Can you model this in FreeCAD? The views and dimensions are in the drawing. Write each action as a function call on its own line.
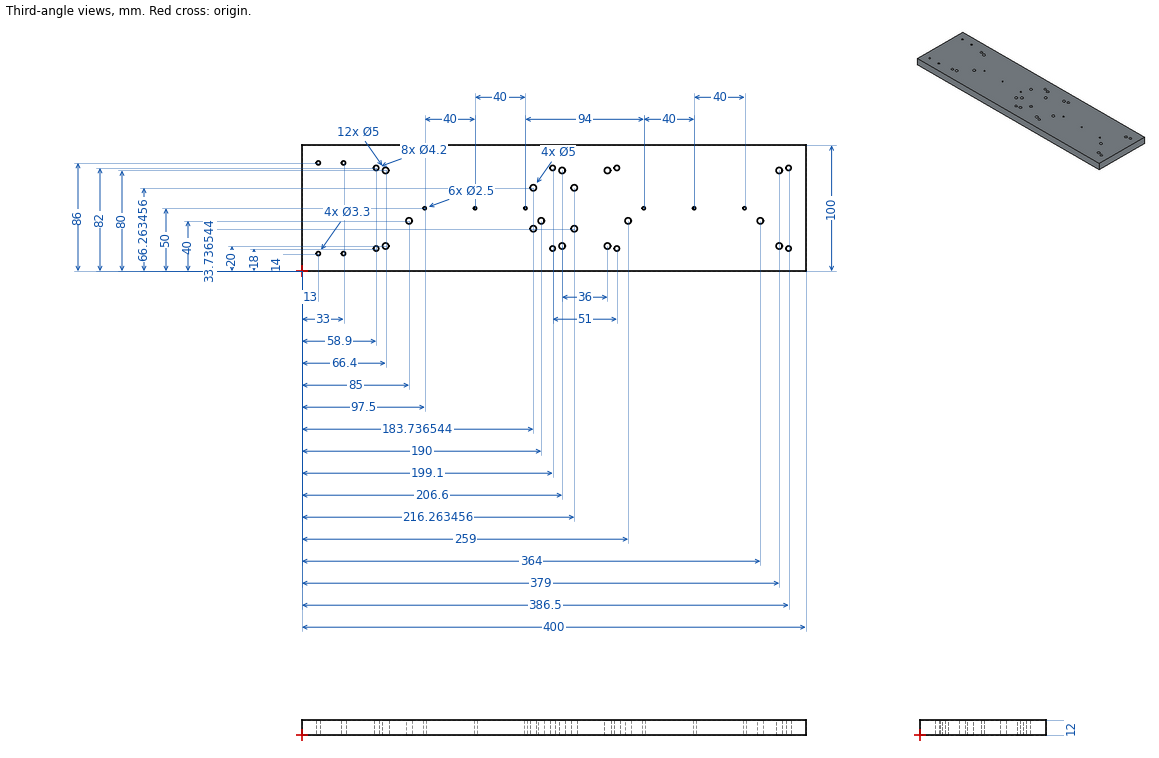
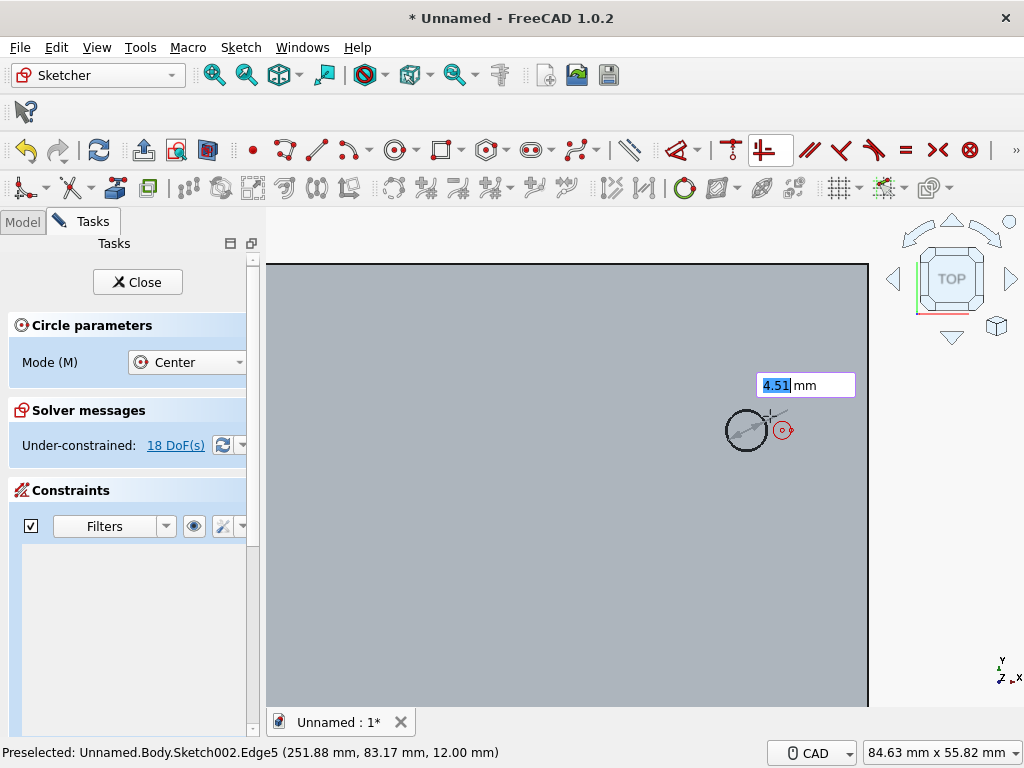
click(761, 411)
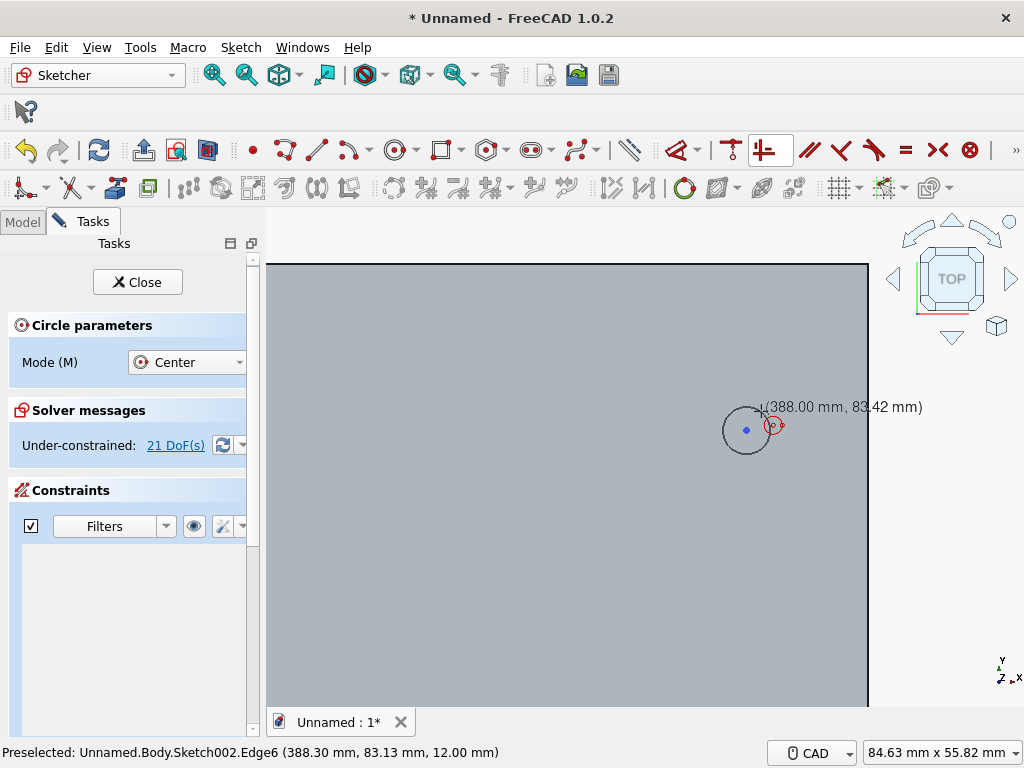
scroll(770, 416, down, 11)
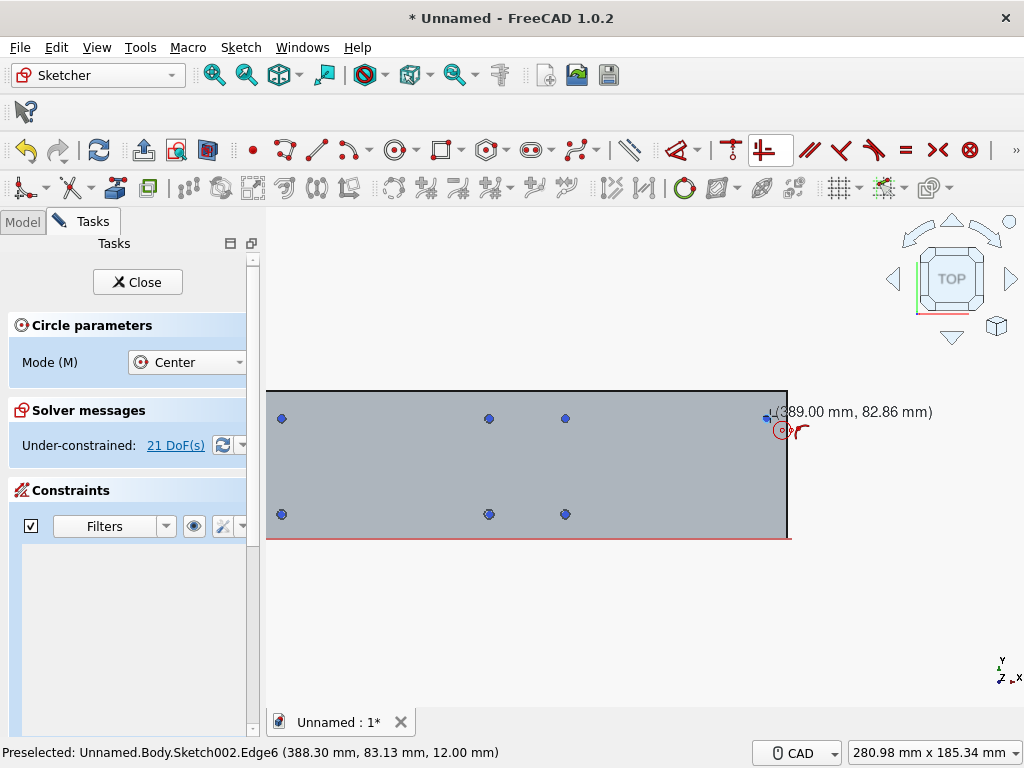
scroll(768, 481, up, 12)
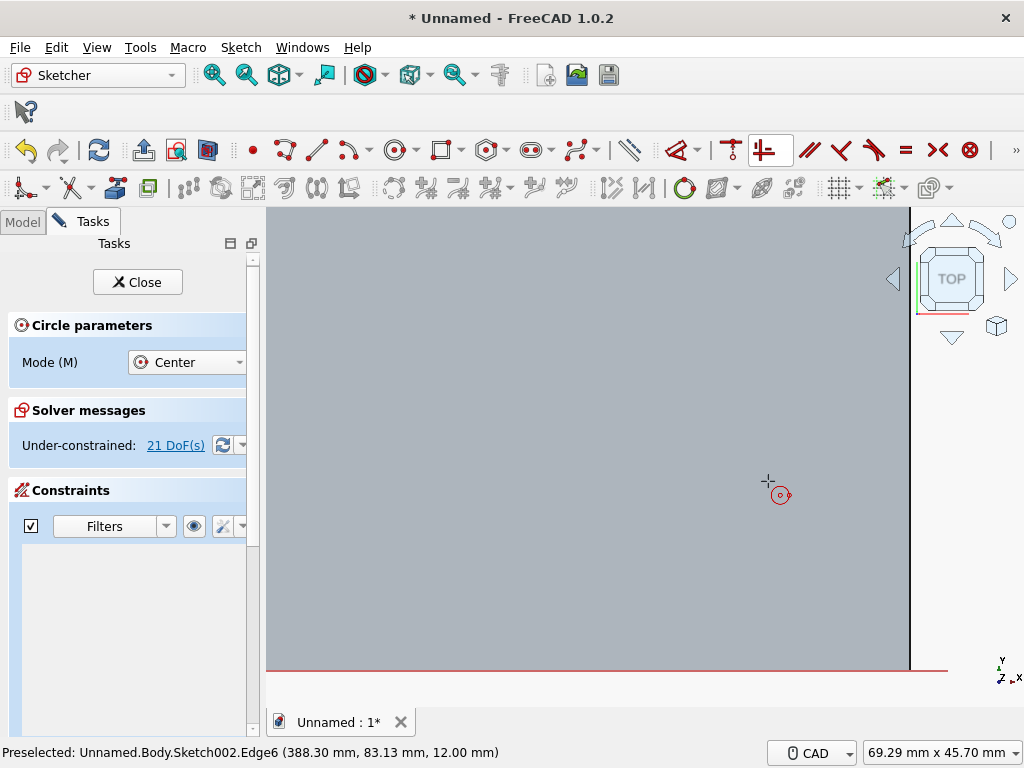
scroll(768, 482, down, 12)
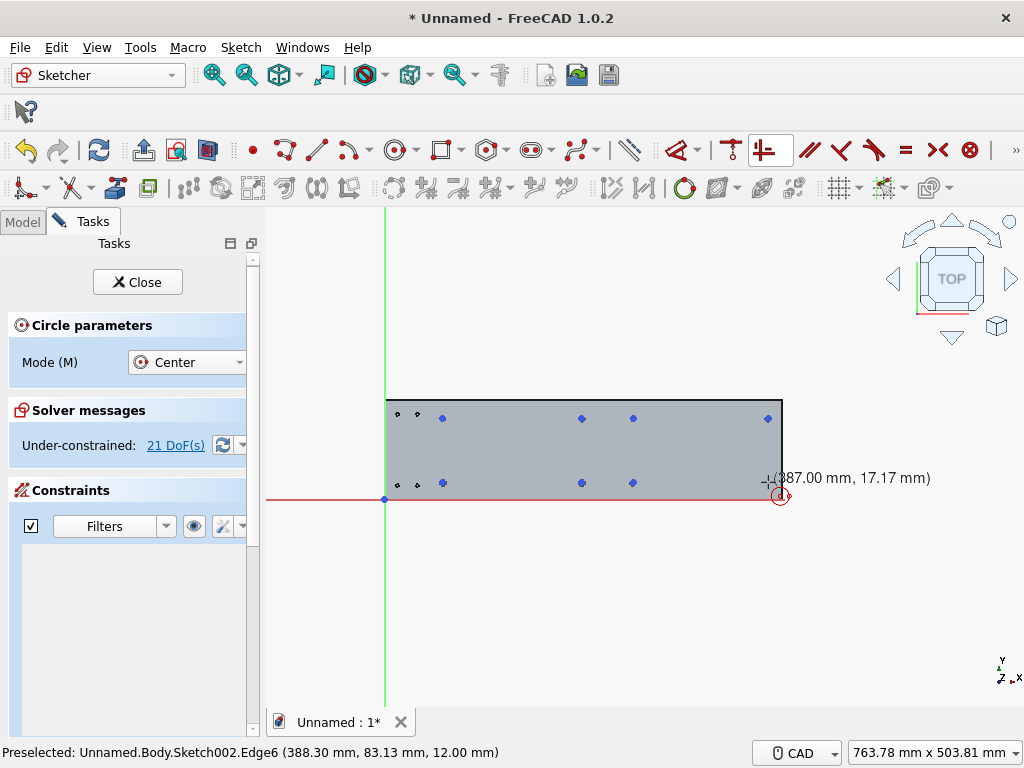
click(768, 482)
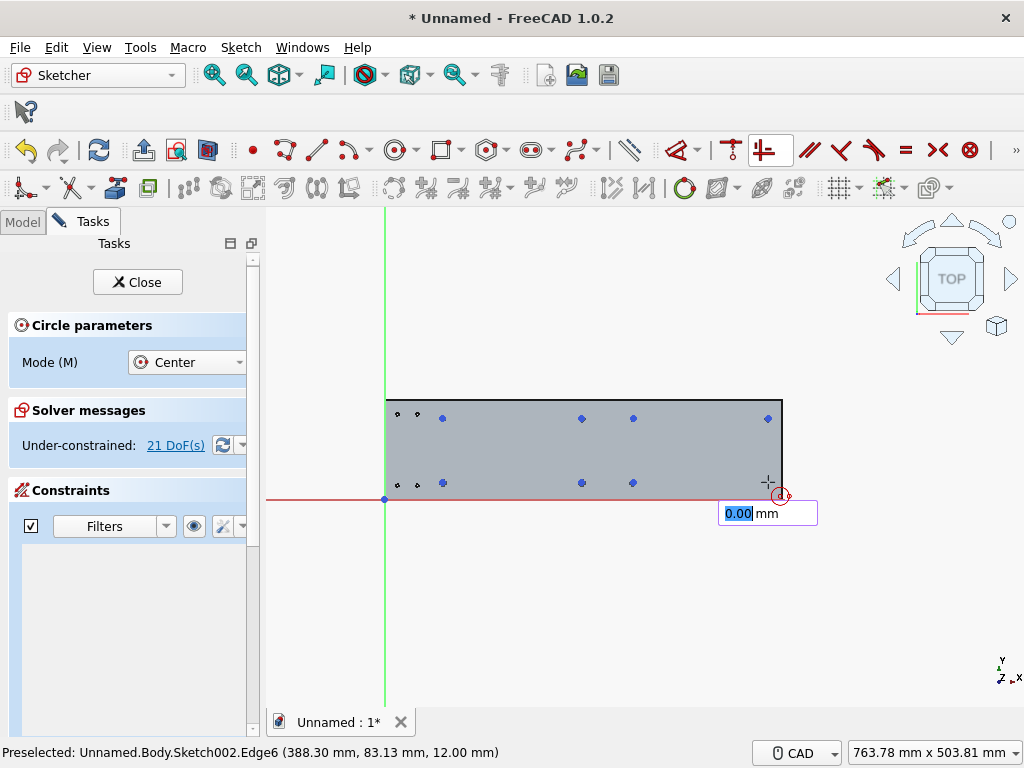
scroll(770, 480, up, 11)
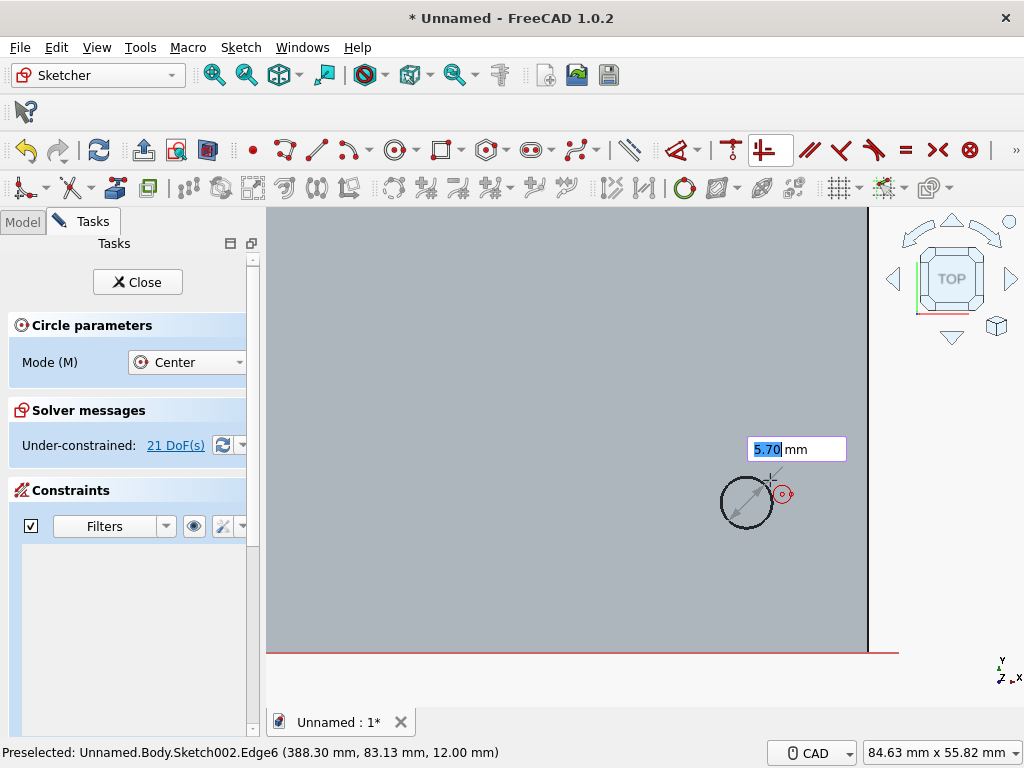
click(761, 478)
key(Escape)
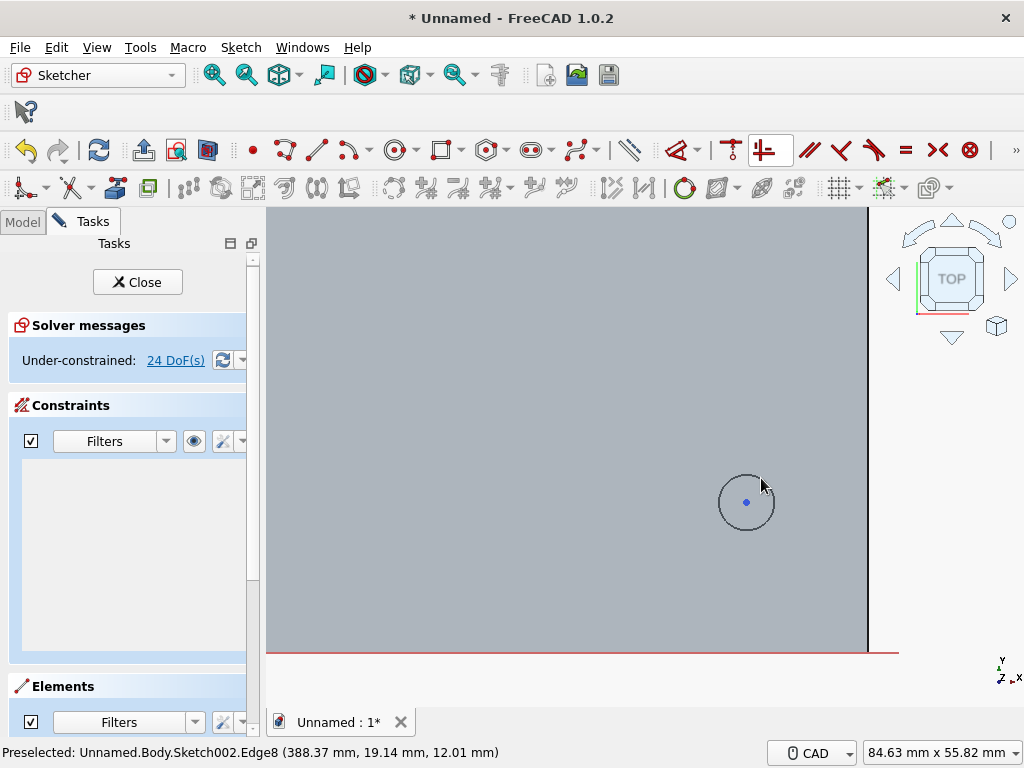
scroll(770, 480, down, 11)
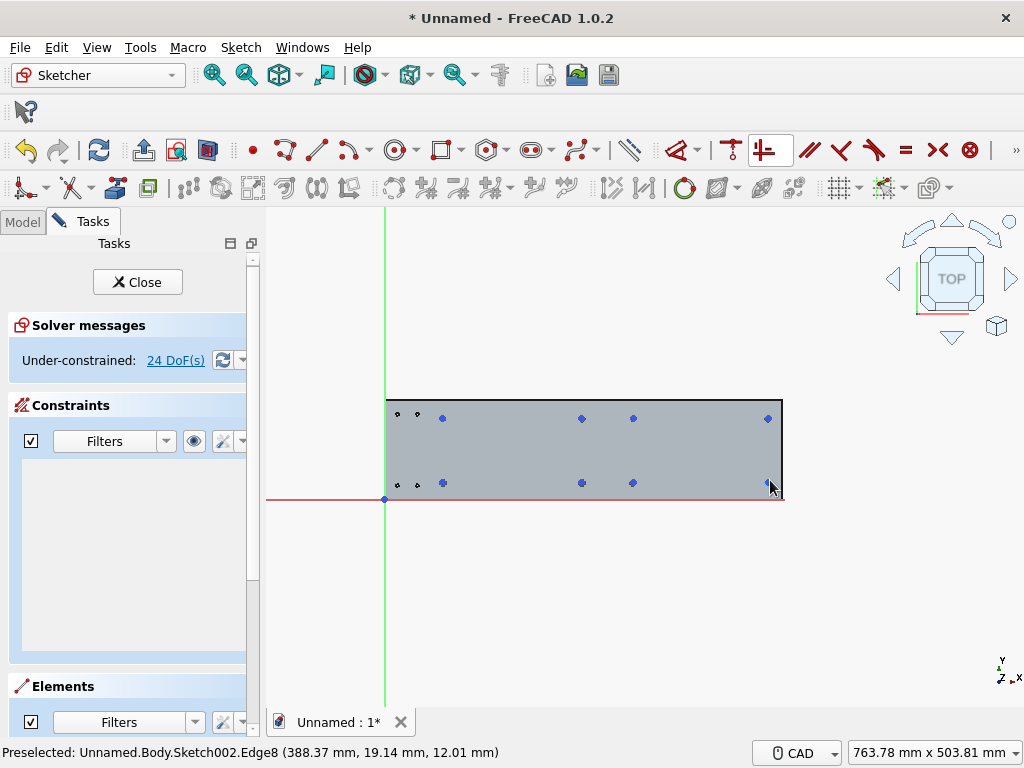
scroll(445, 417, up, 9)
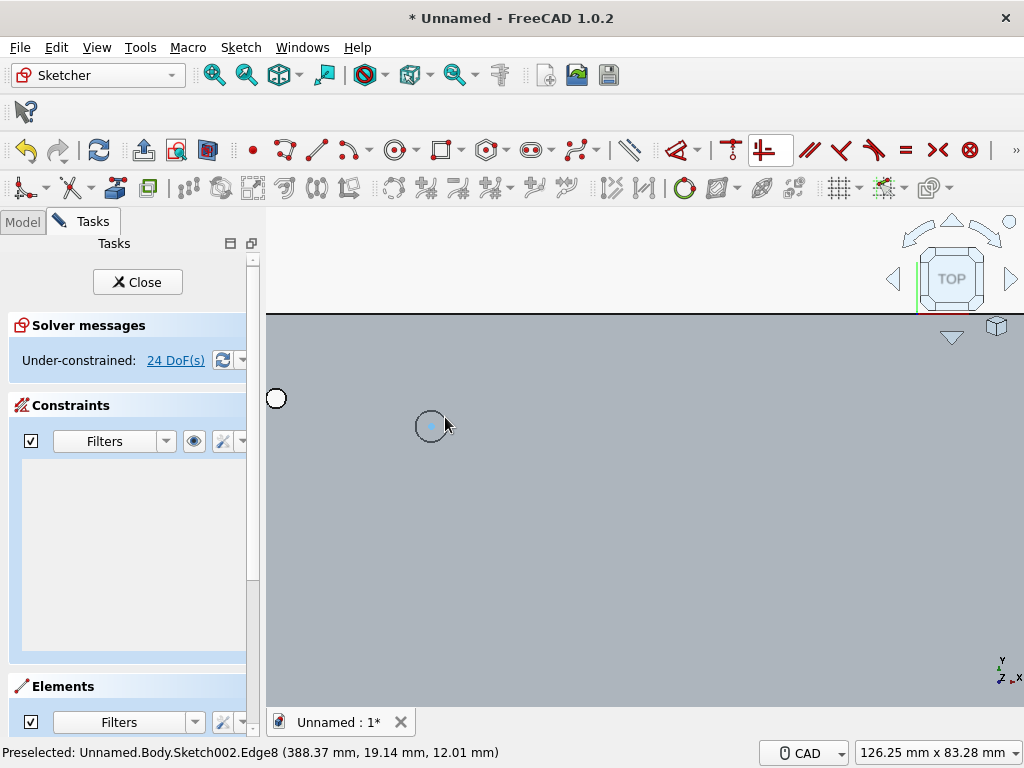
click(442, 415)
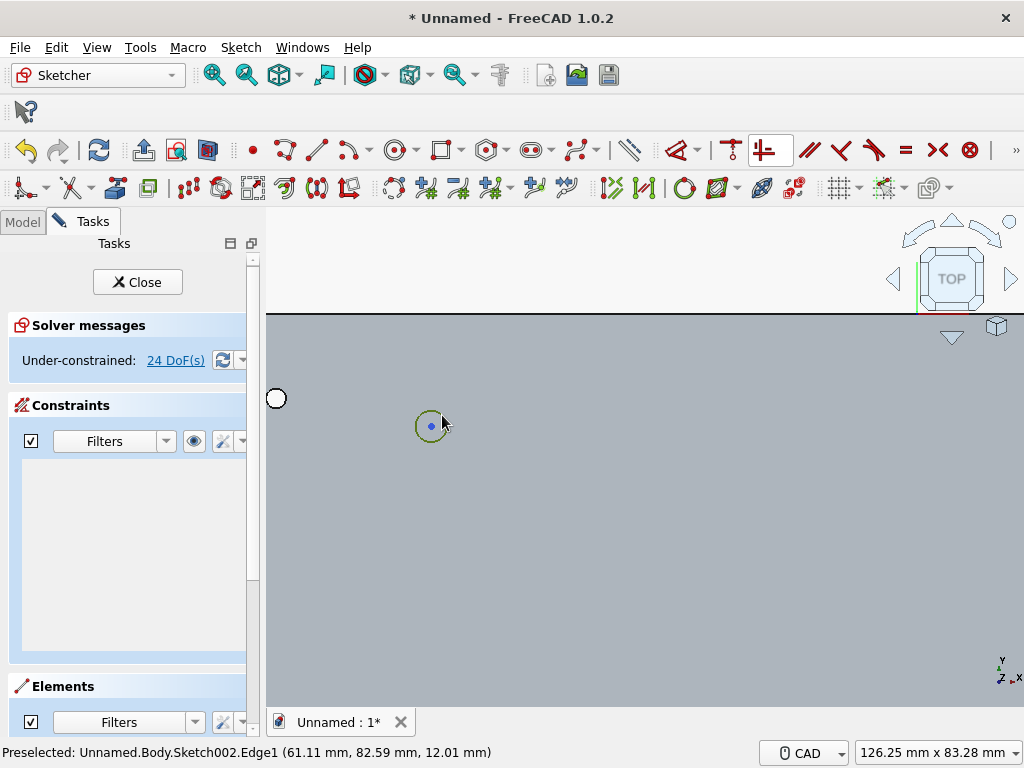
scroll(444, 416, down, 9)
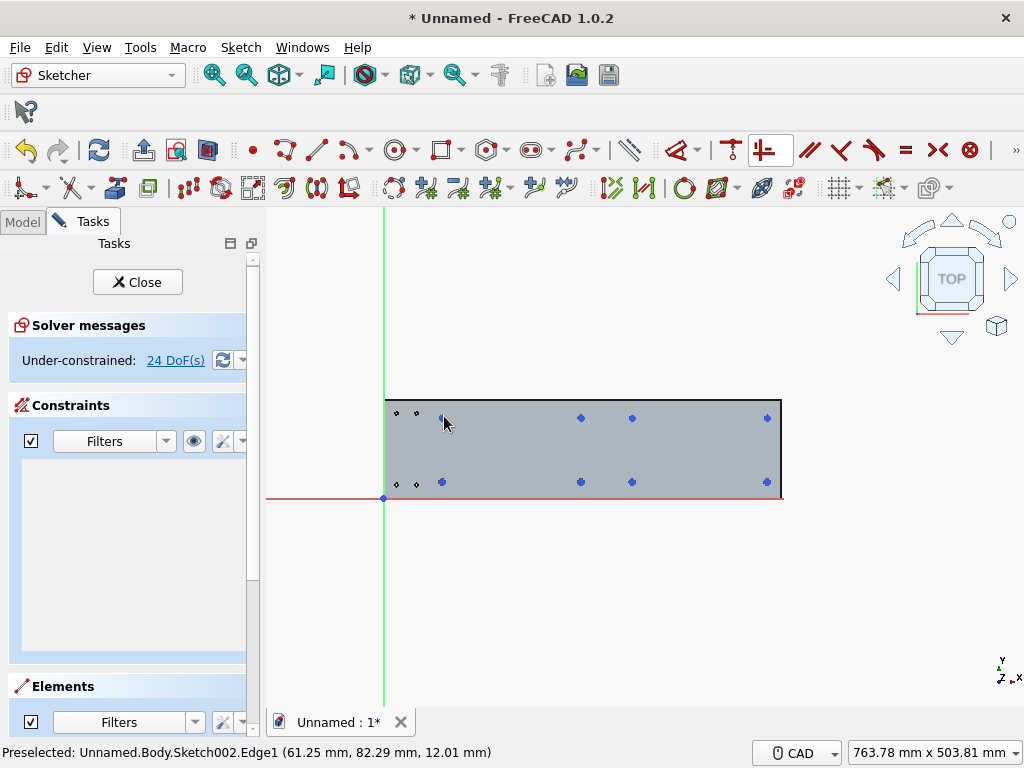
scroll(444, 480, up, 8)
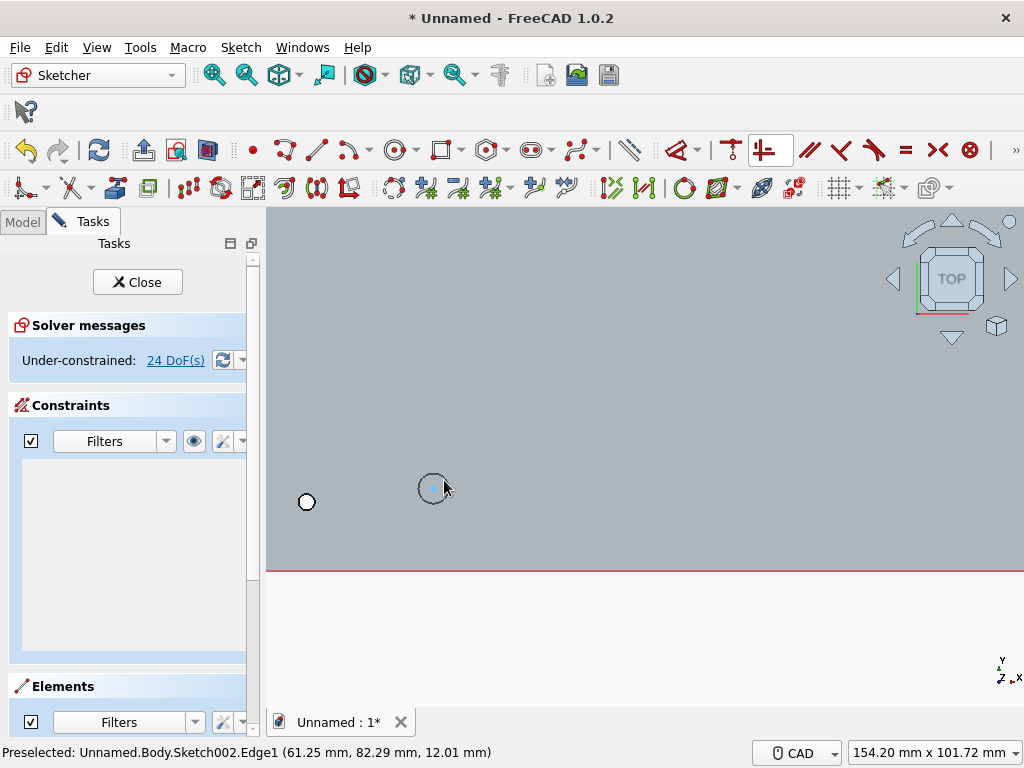
click(444, 478)